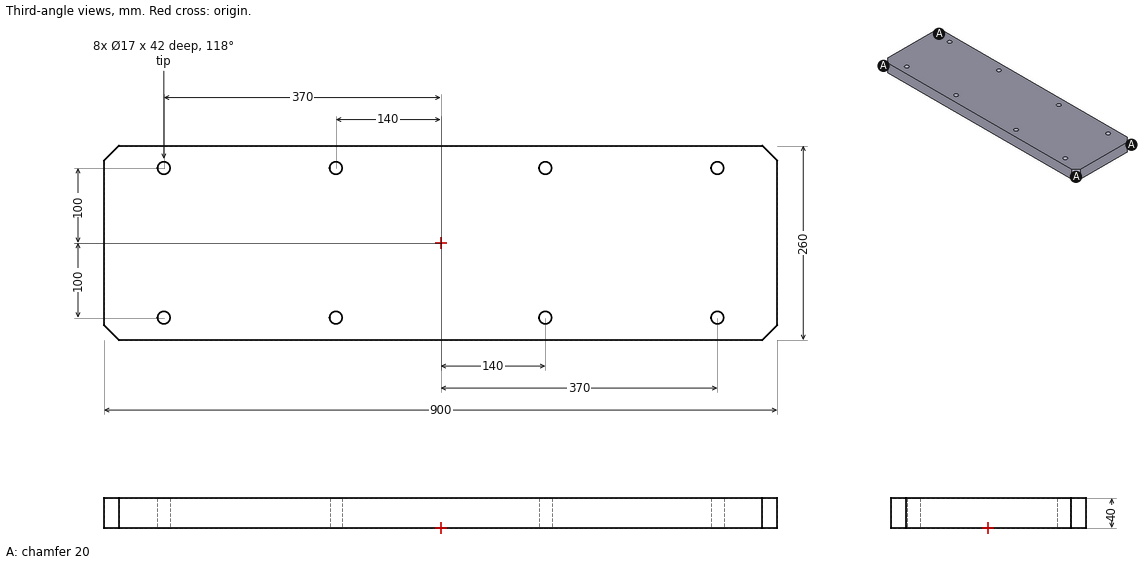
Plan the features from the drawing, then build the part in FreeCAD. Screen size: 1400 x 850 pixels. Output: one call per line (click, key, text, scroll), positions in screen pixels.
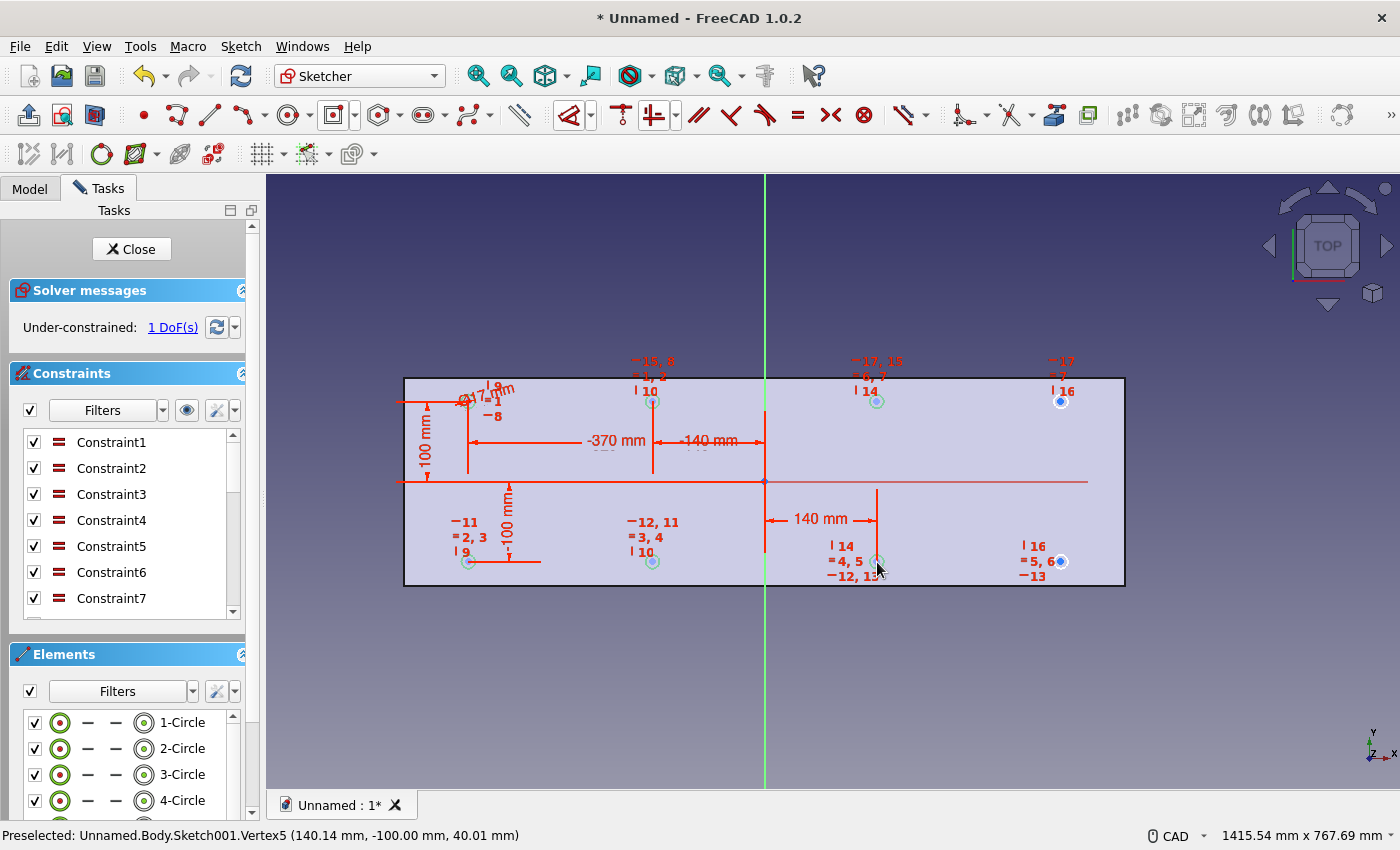
click(1061, 562)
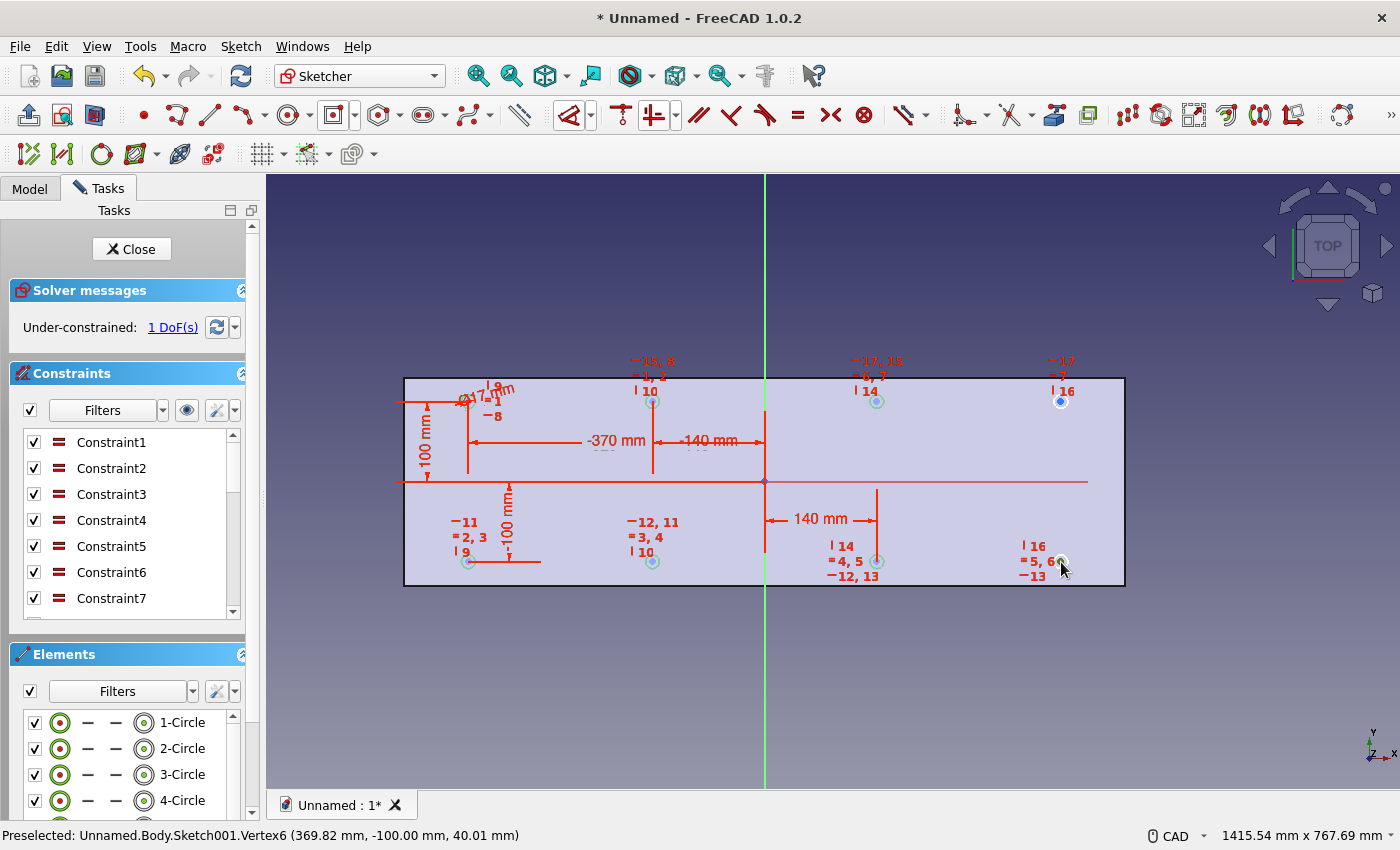
key(l)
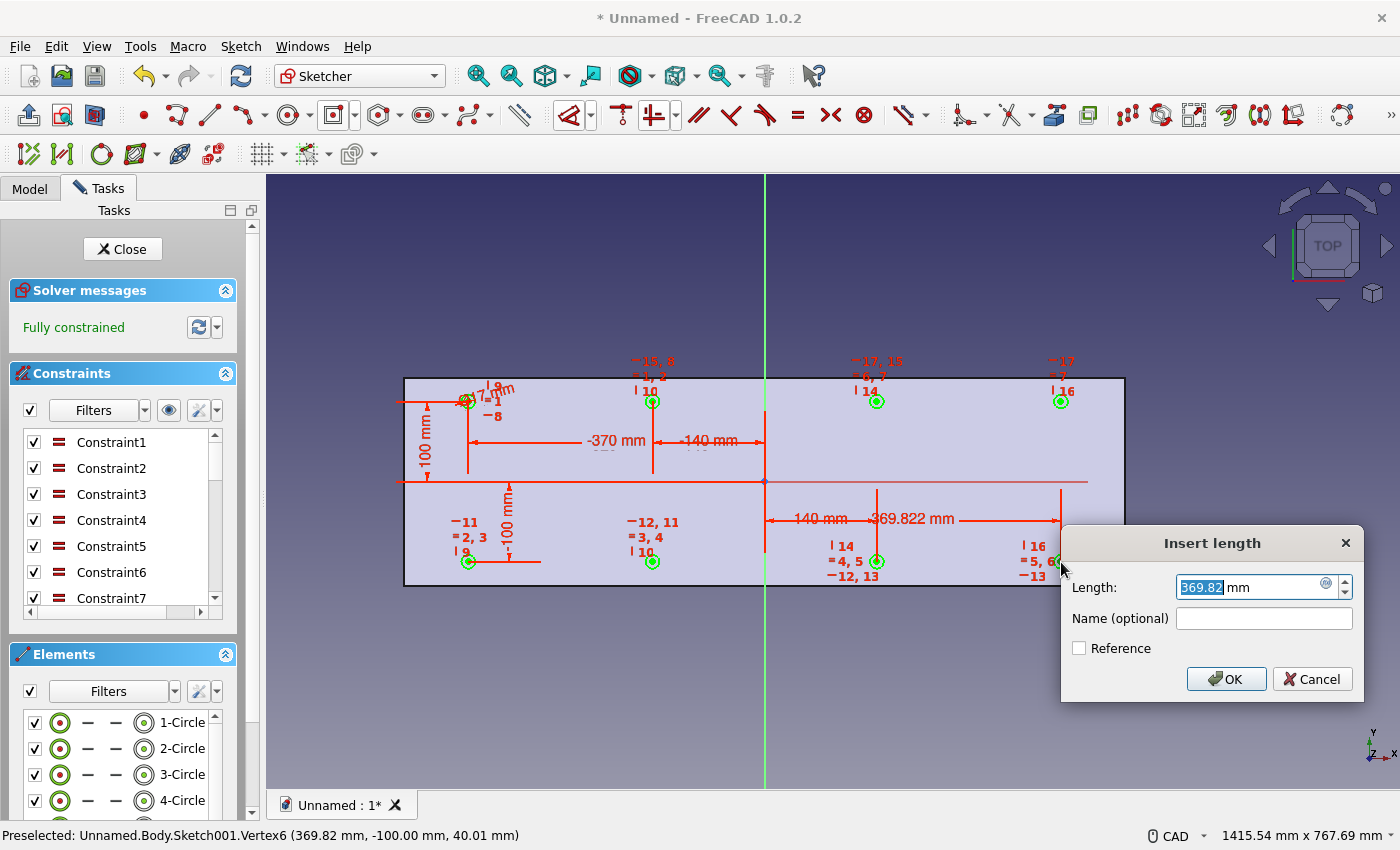
text(370)
key(Return)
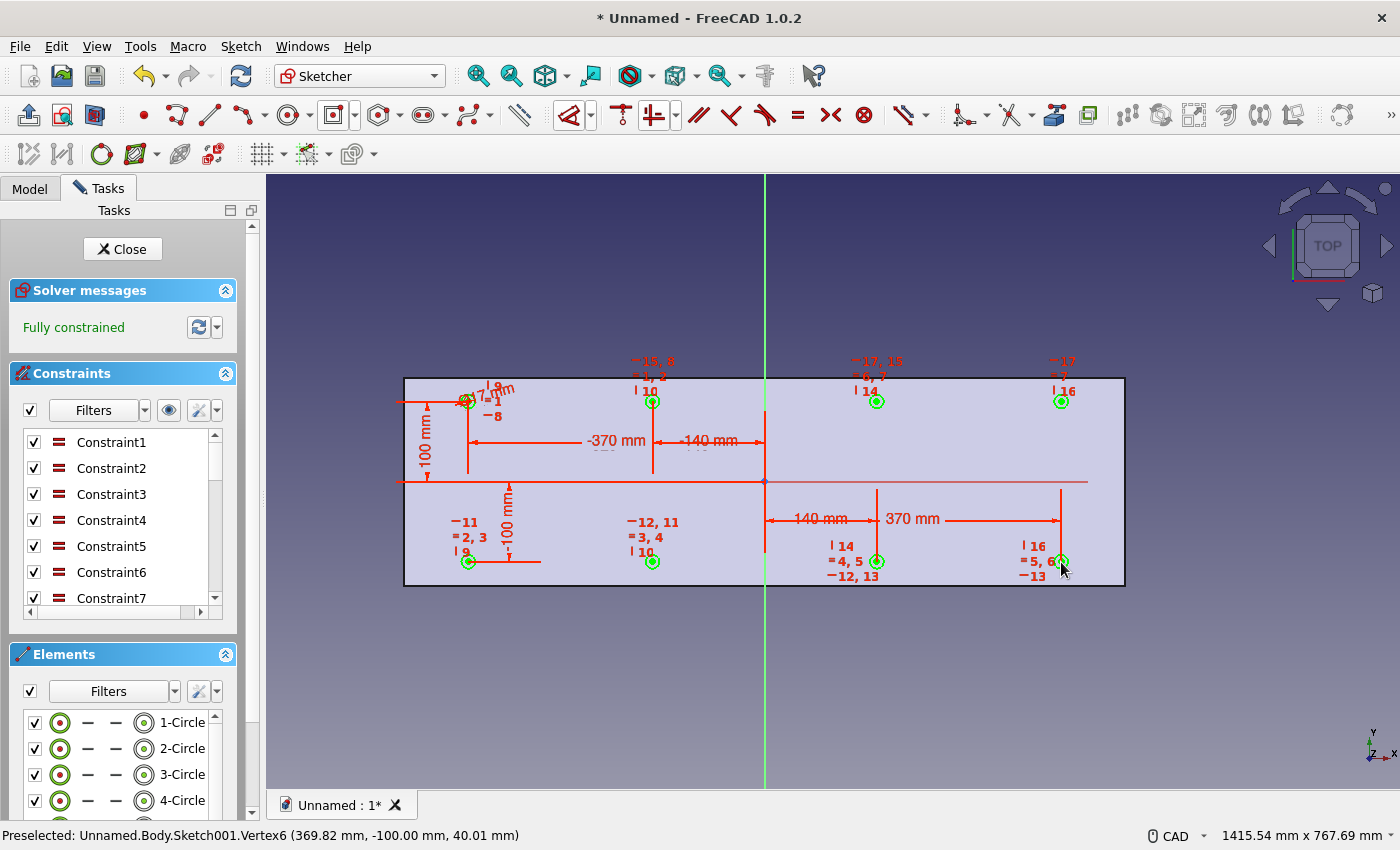
click(123, 249)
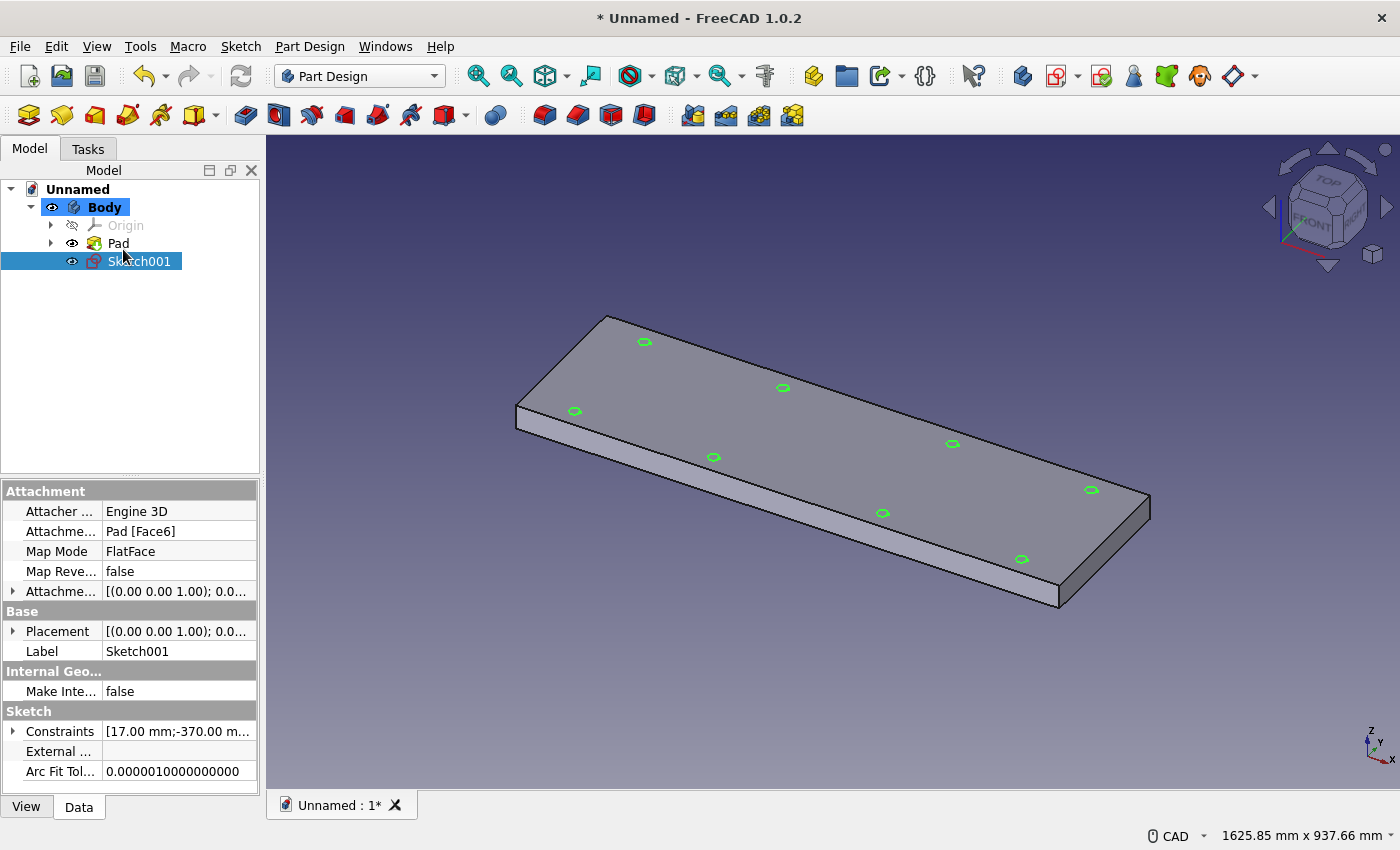
click(279, 116)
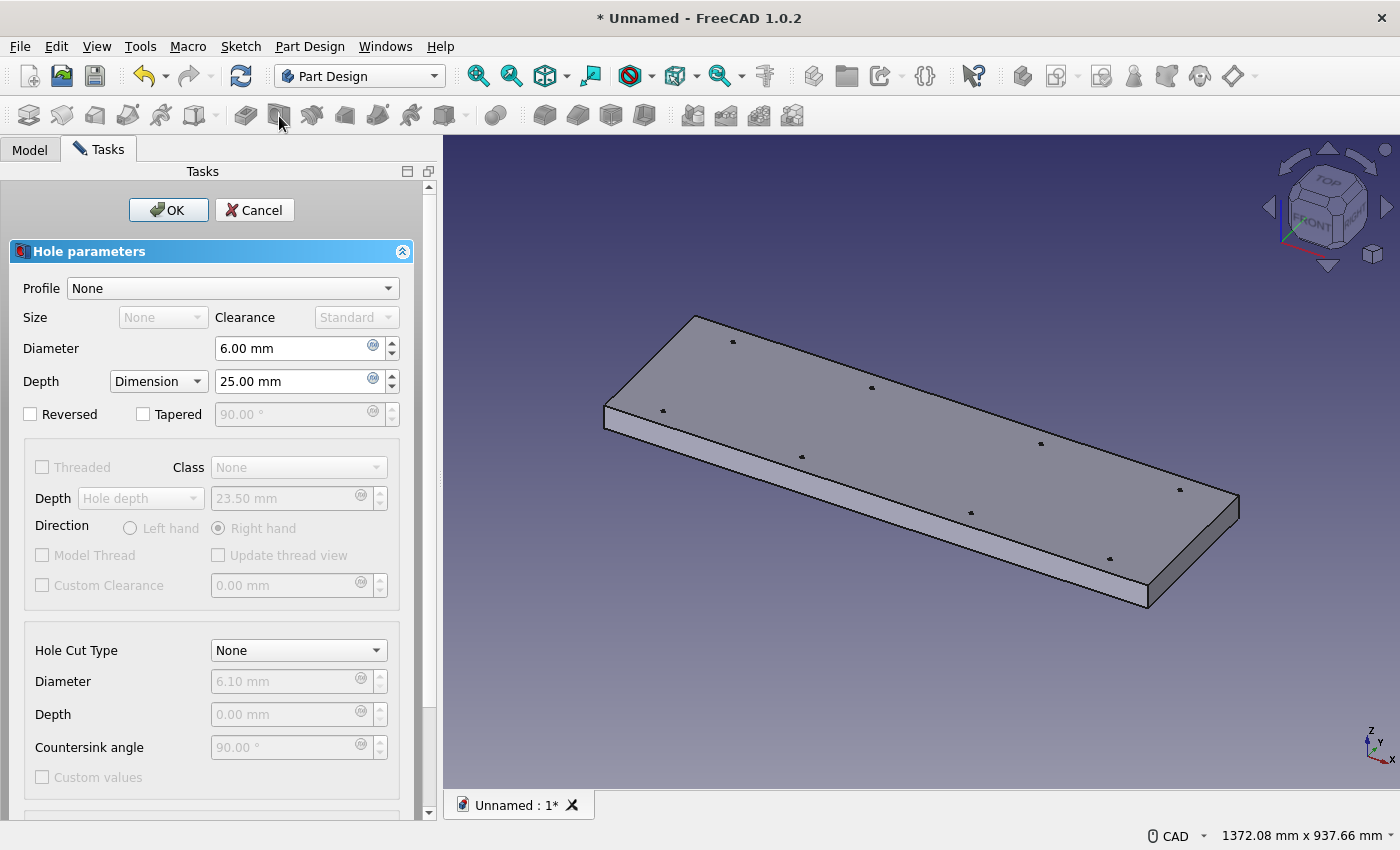
triple_click(300, 348)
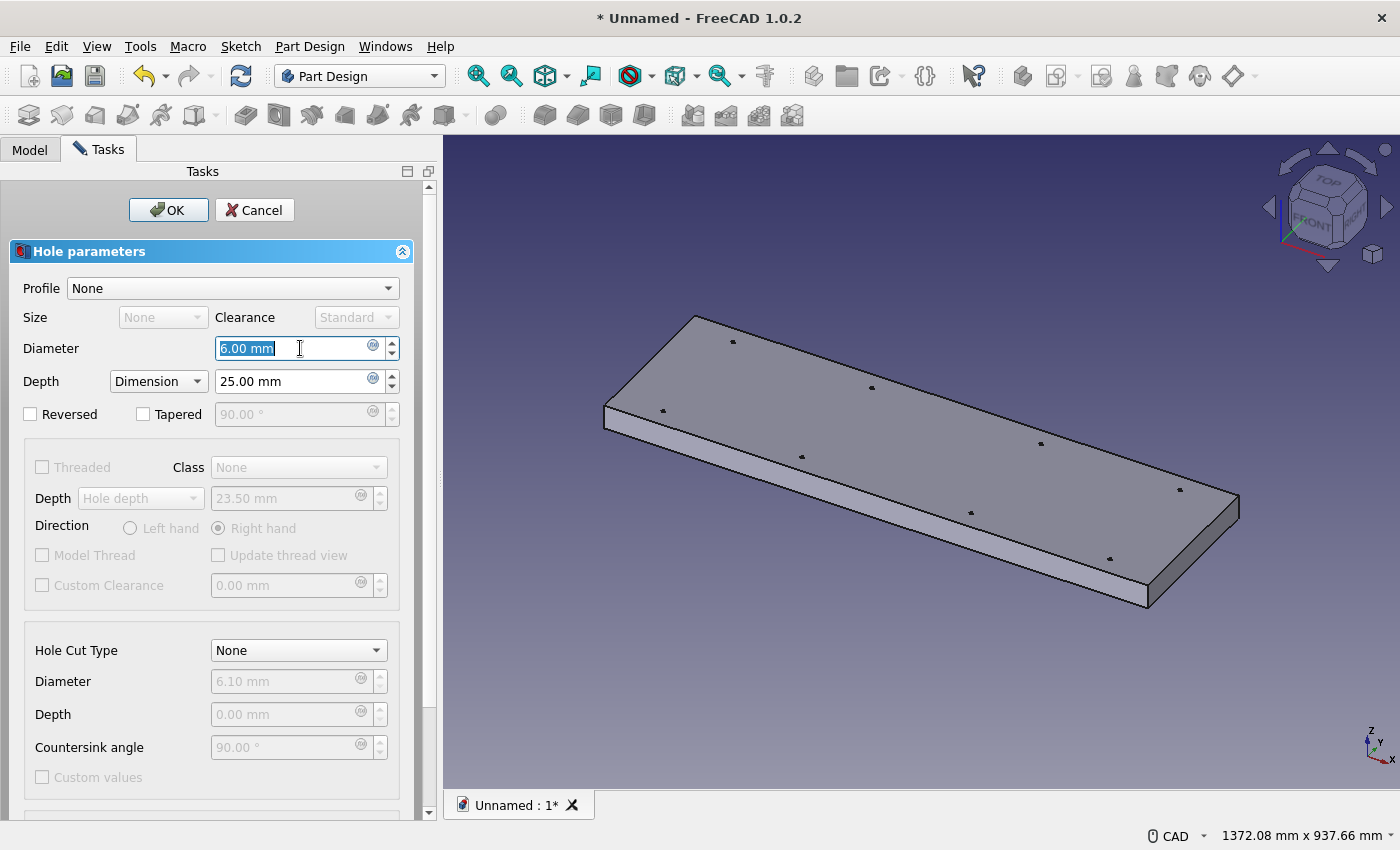
text(17)
key(Tab)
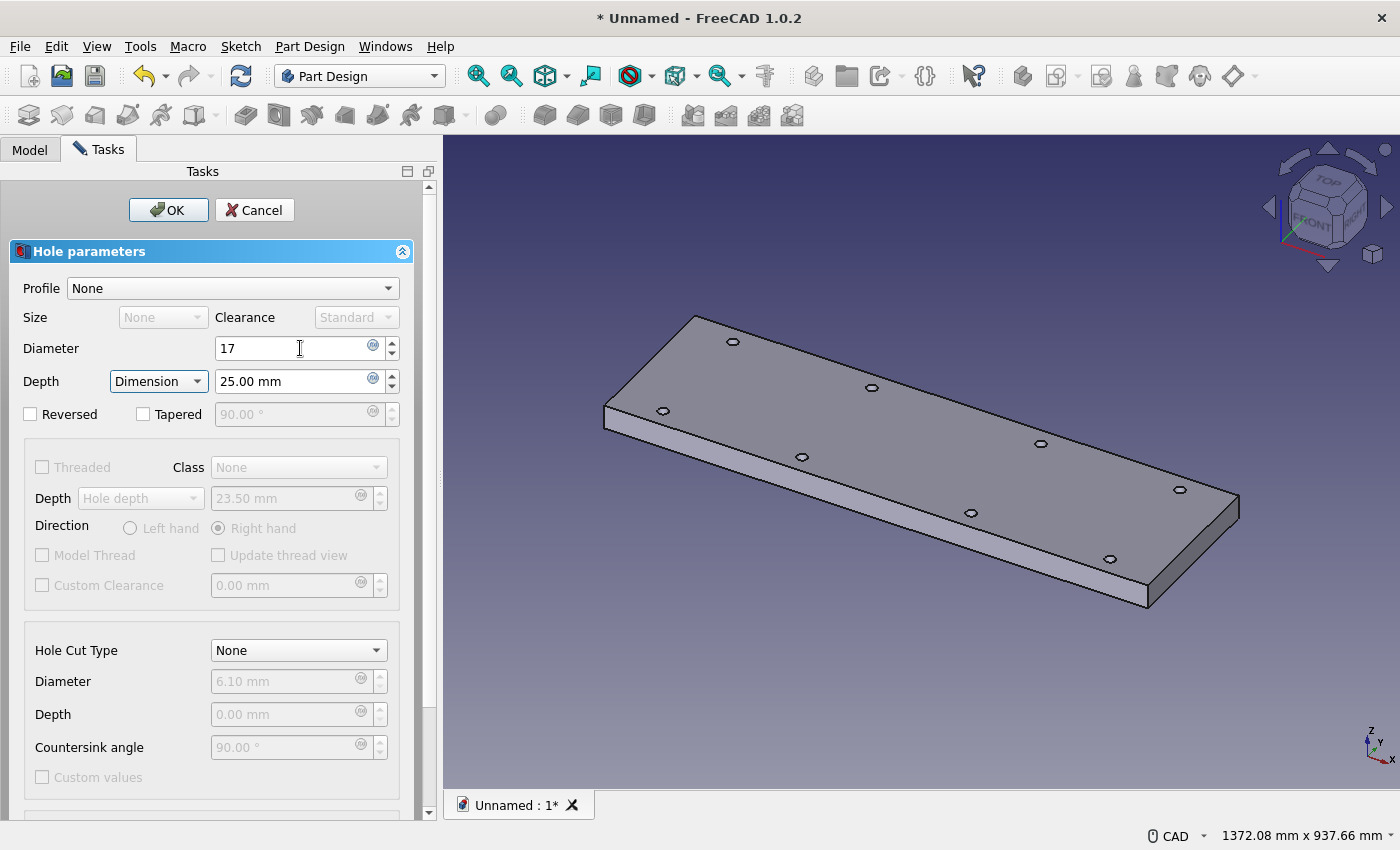
triple_click(300, 382)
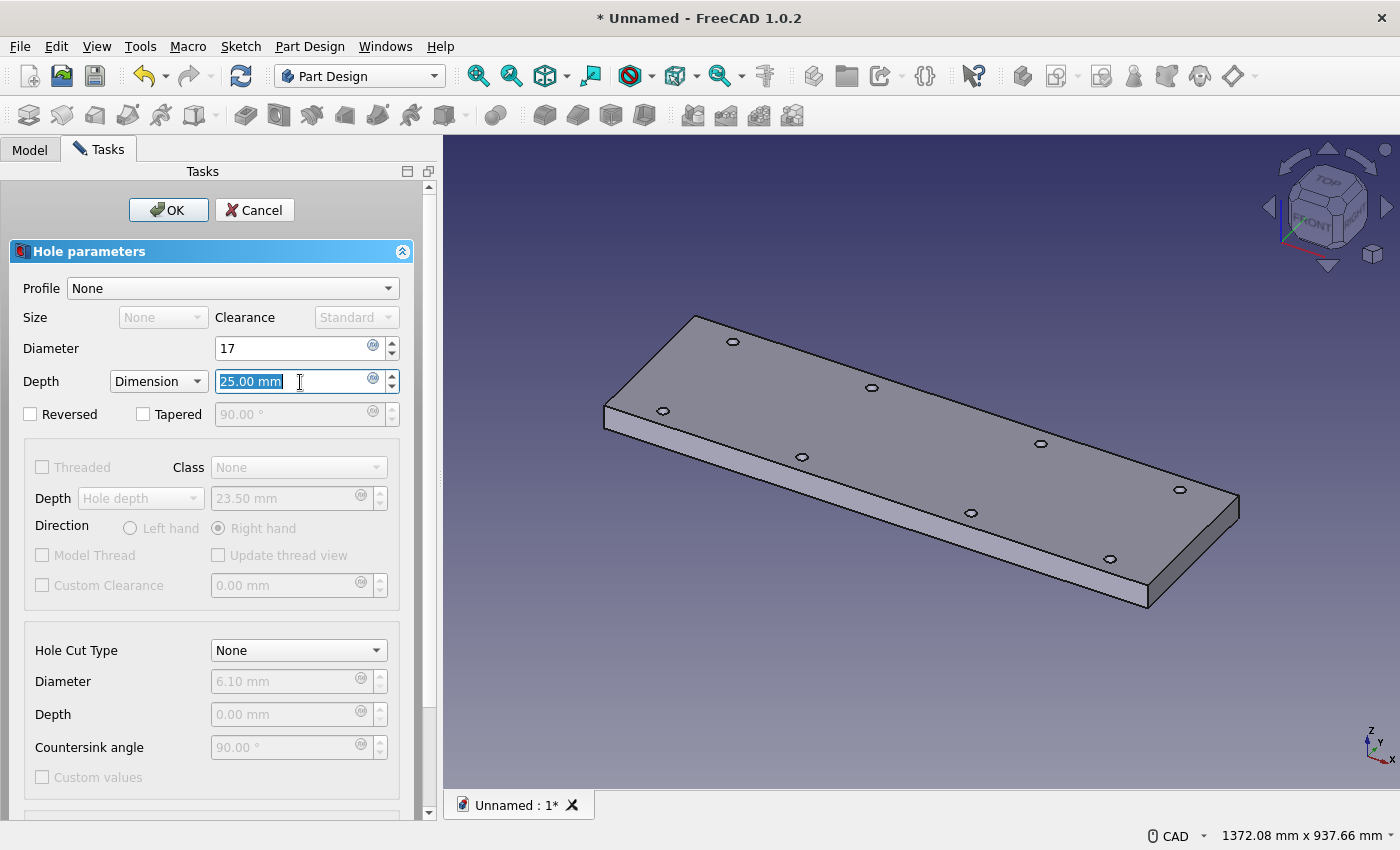
text(42)
key(Tab)